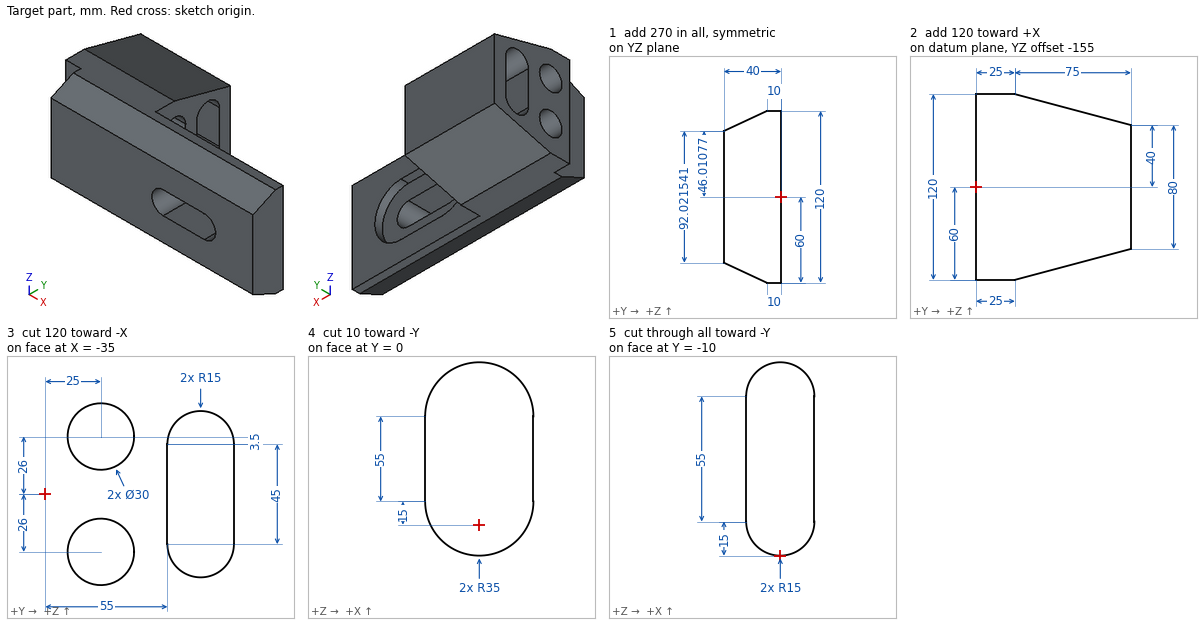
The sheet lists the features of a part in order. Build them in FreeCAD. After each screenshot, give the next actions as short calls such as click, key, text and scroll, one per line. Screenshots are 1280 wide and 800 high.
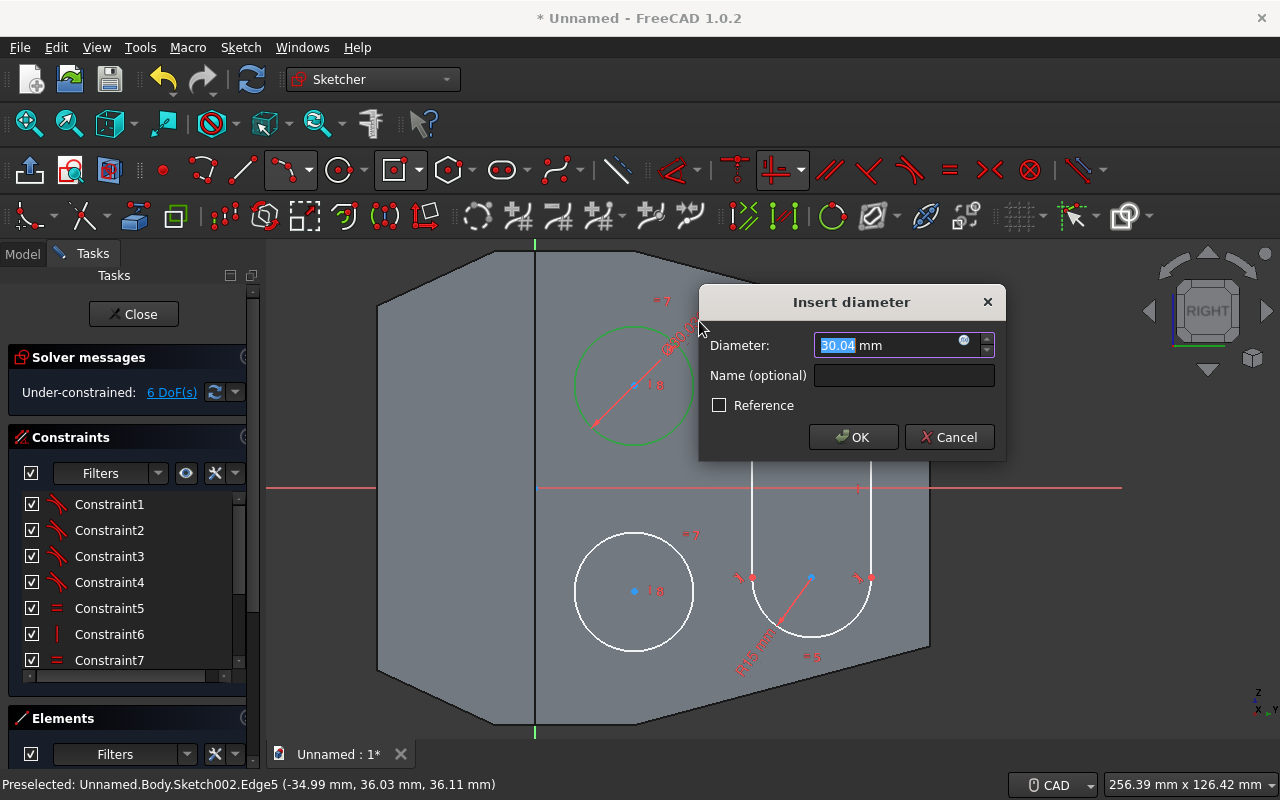
text(30)
key(Return)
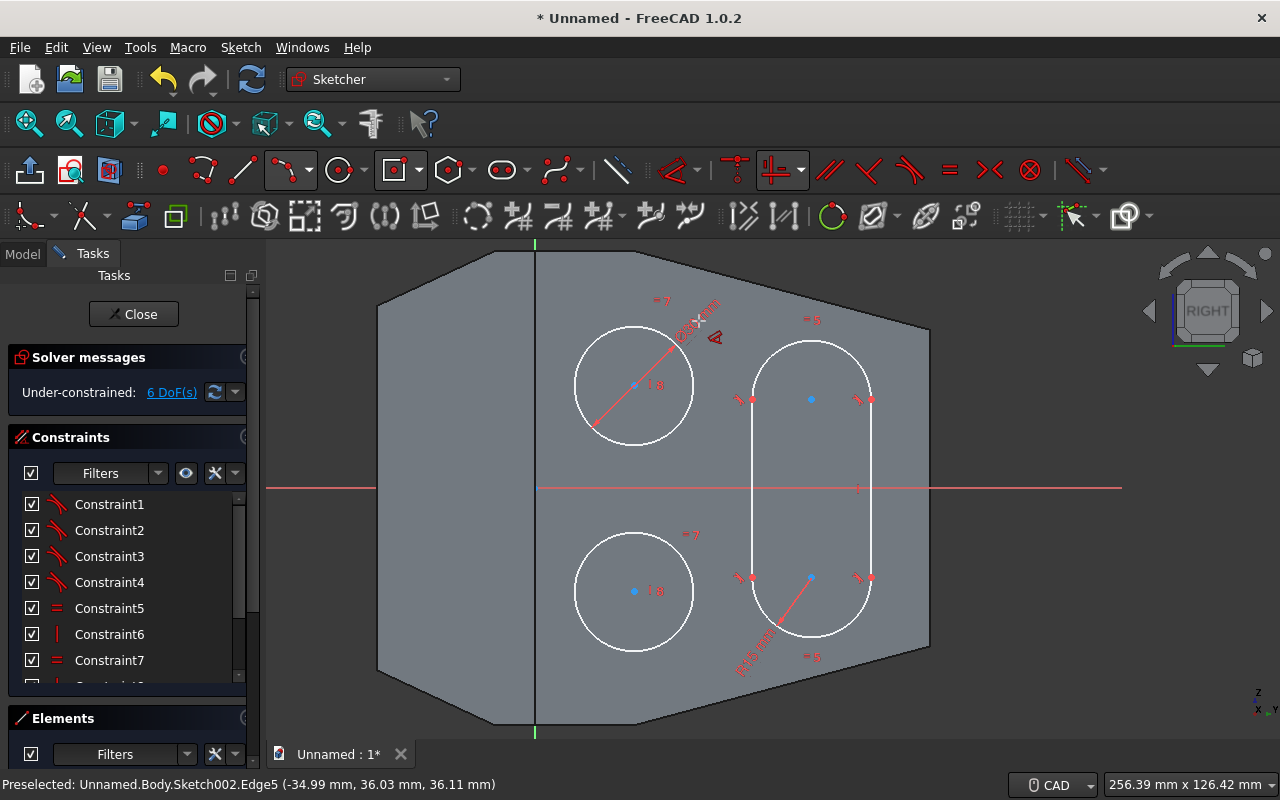
click(752, 525)
click(786, 448)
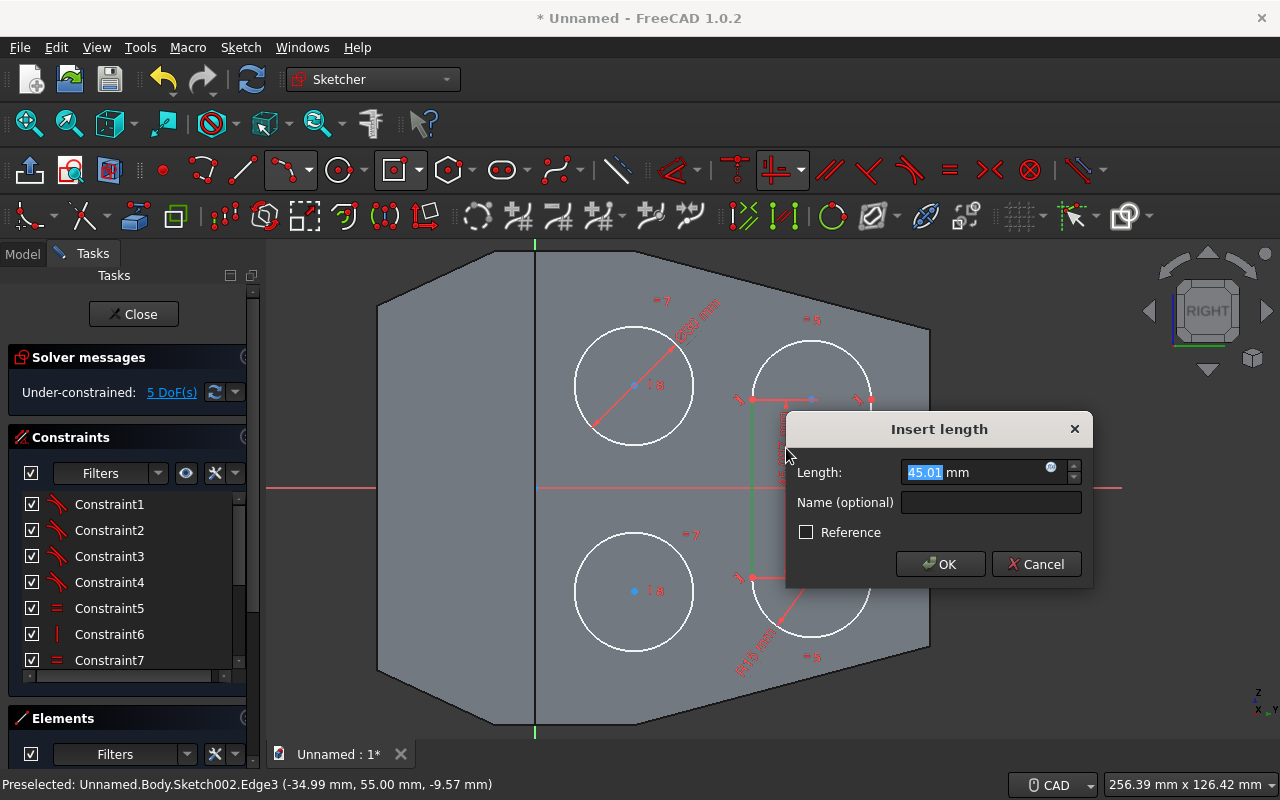
text(45)
key(Return)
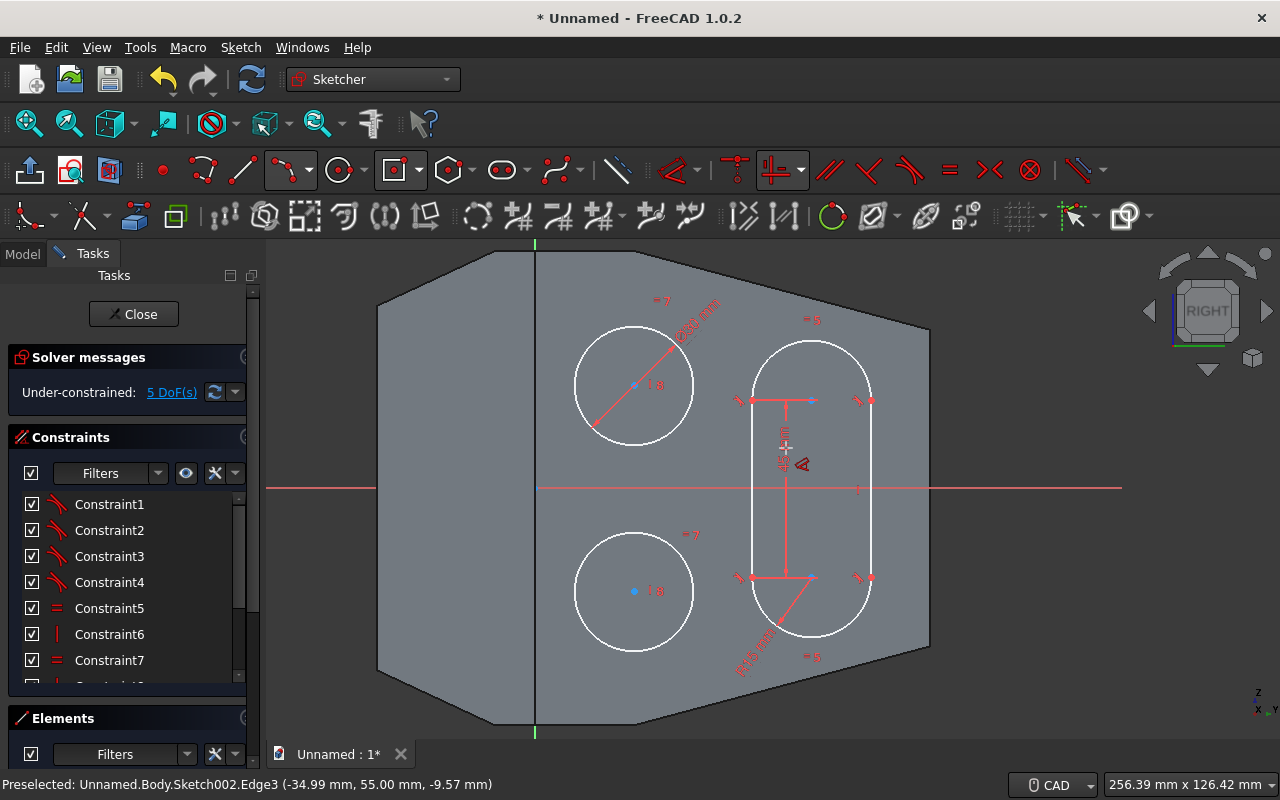
click(634, 386)
click(562, 352)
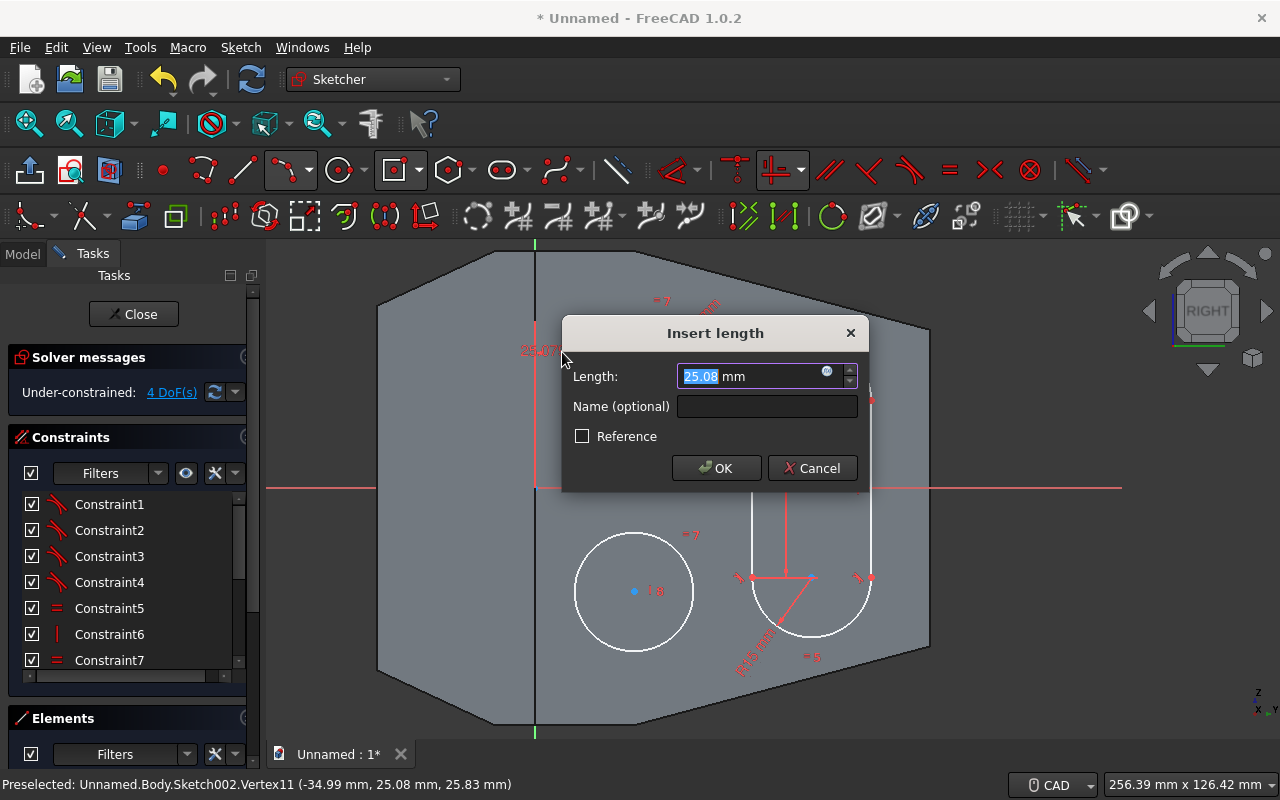
text(25)
key(Return)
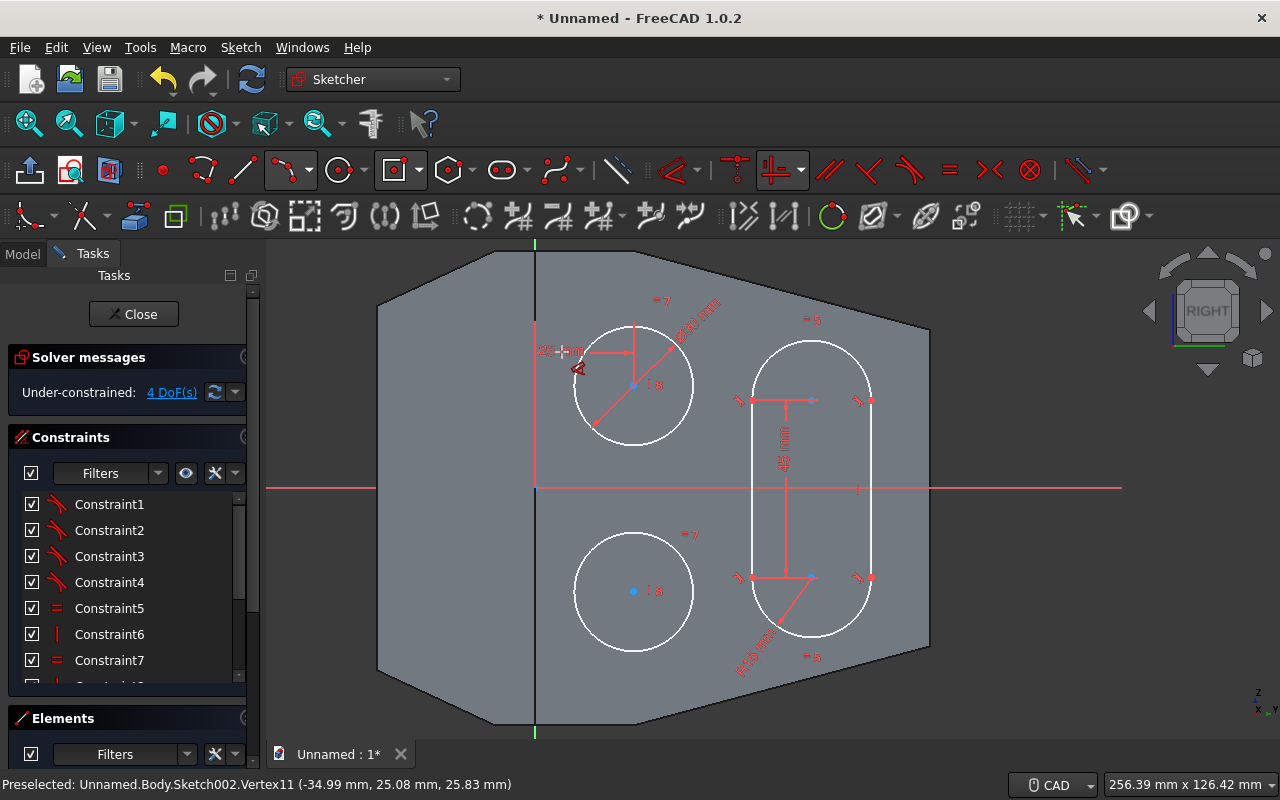
click(634, 386)
click(501, 437)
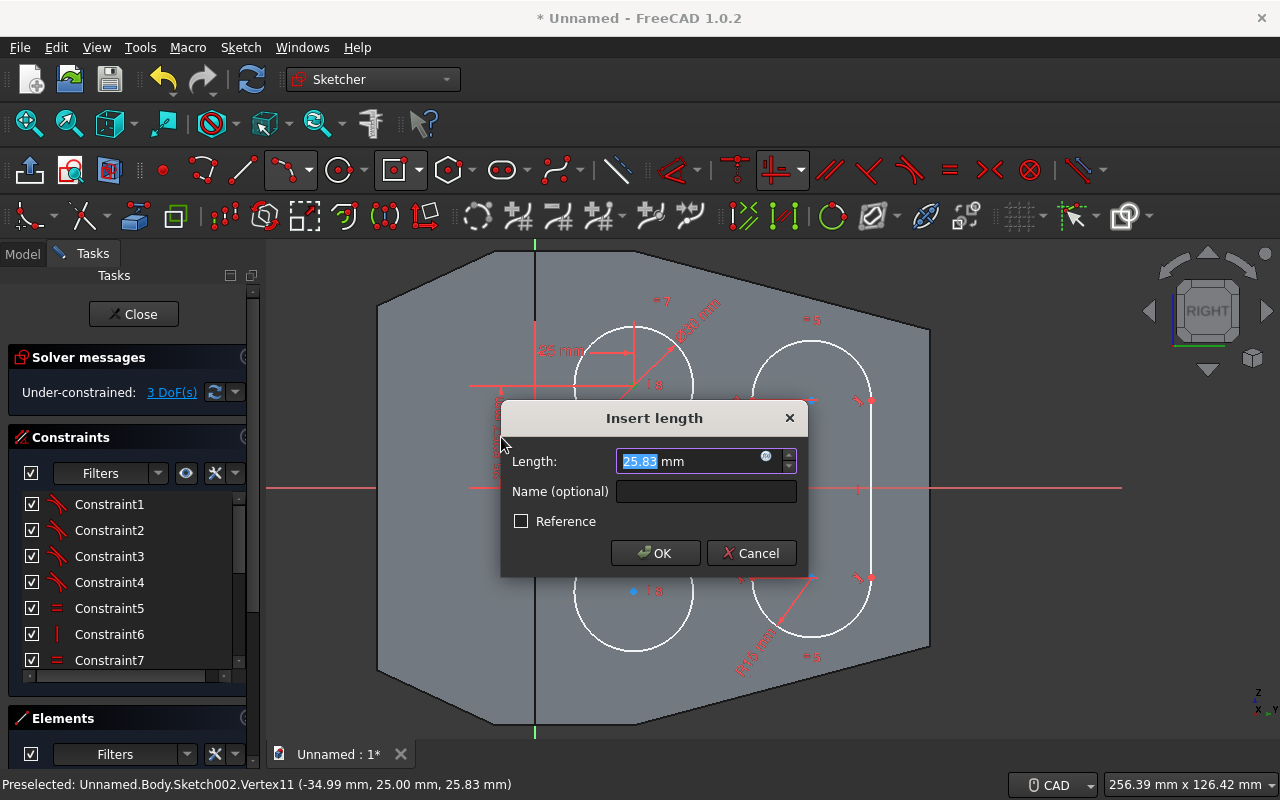
text(26)
key(Return)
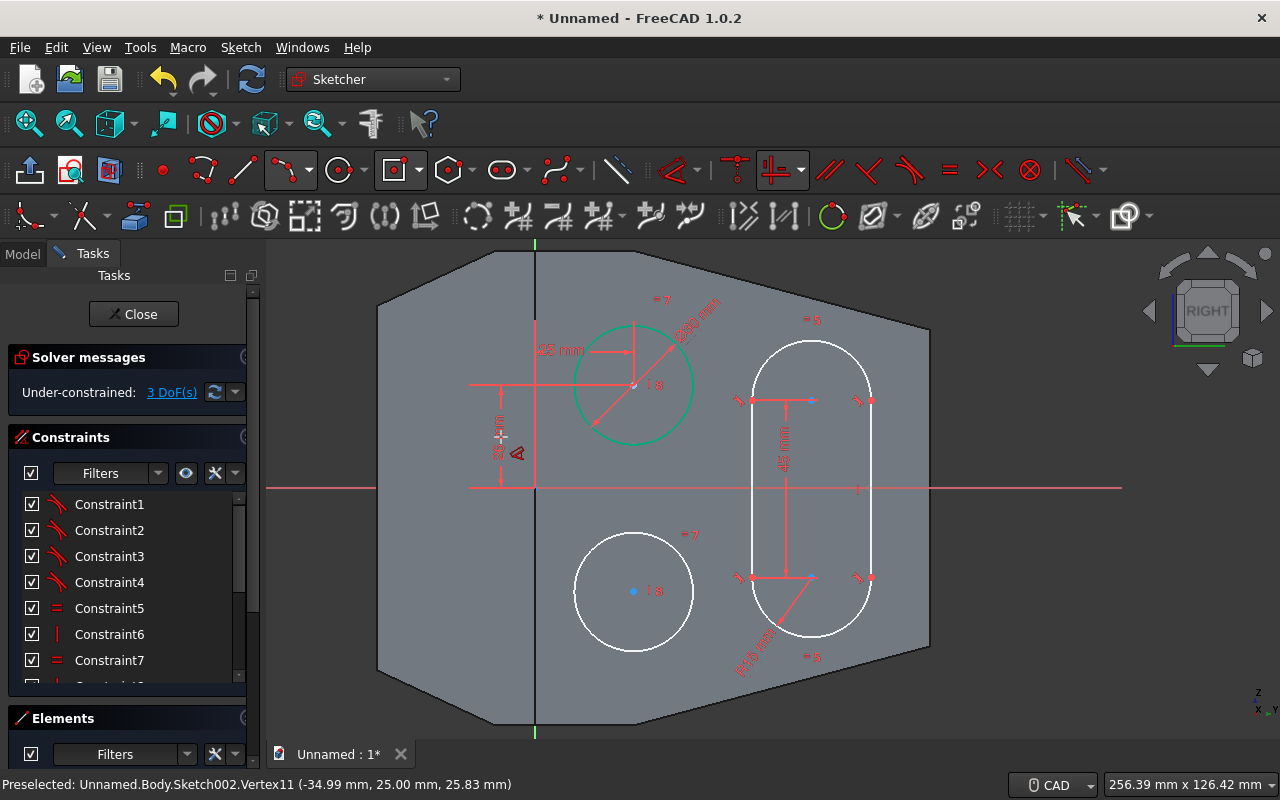
click(634, 592)
click(501, 540)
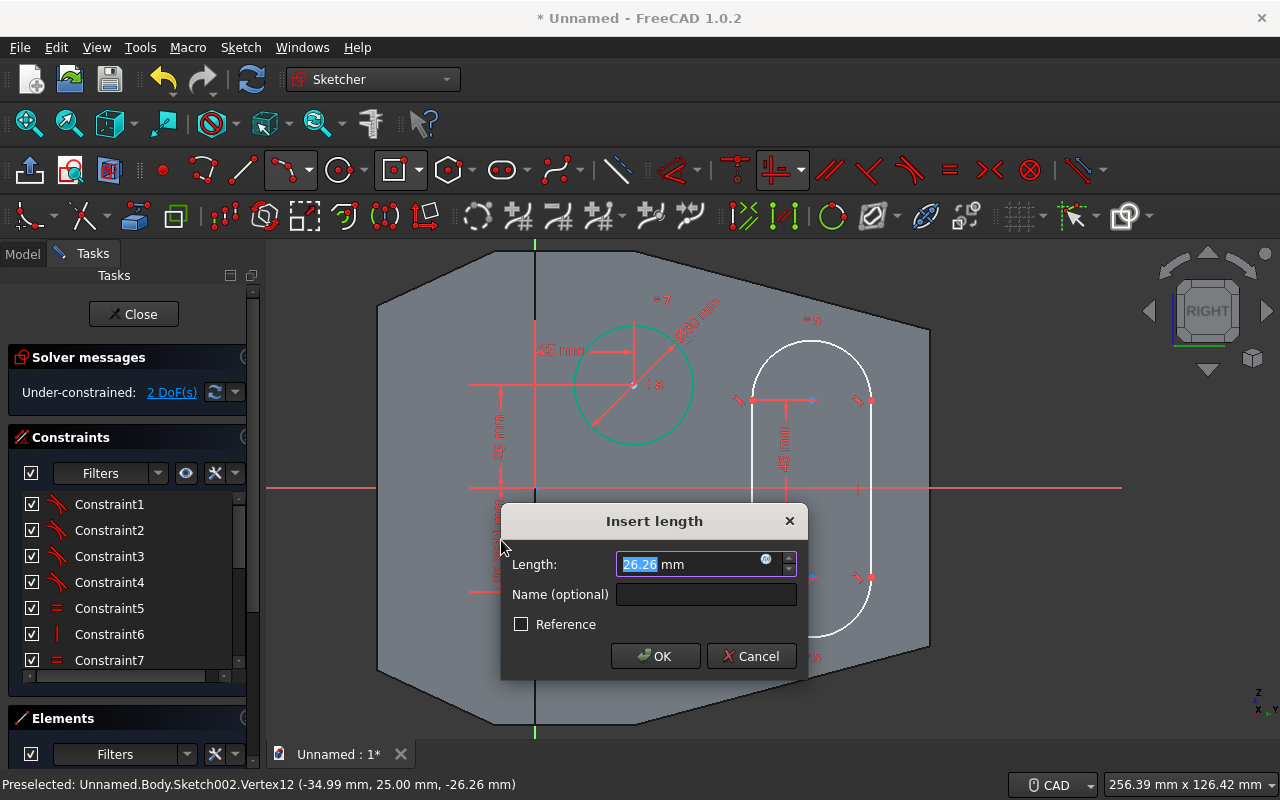
text(26)
key(Return)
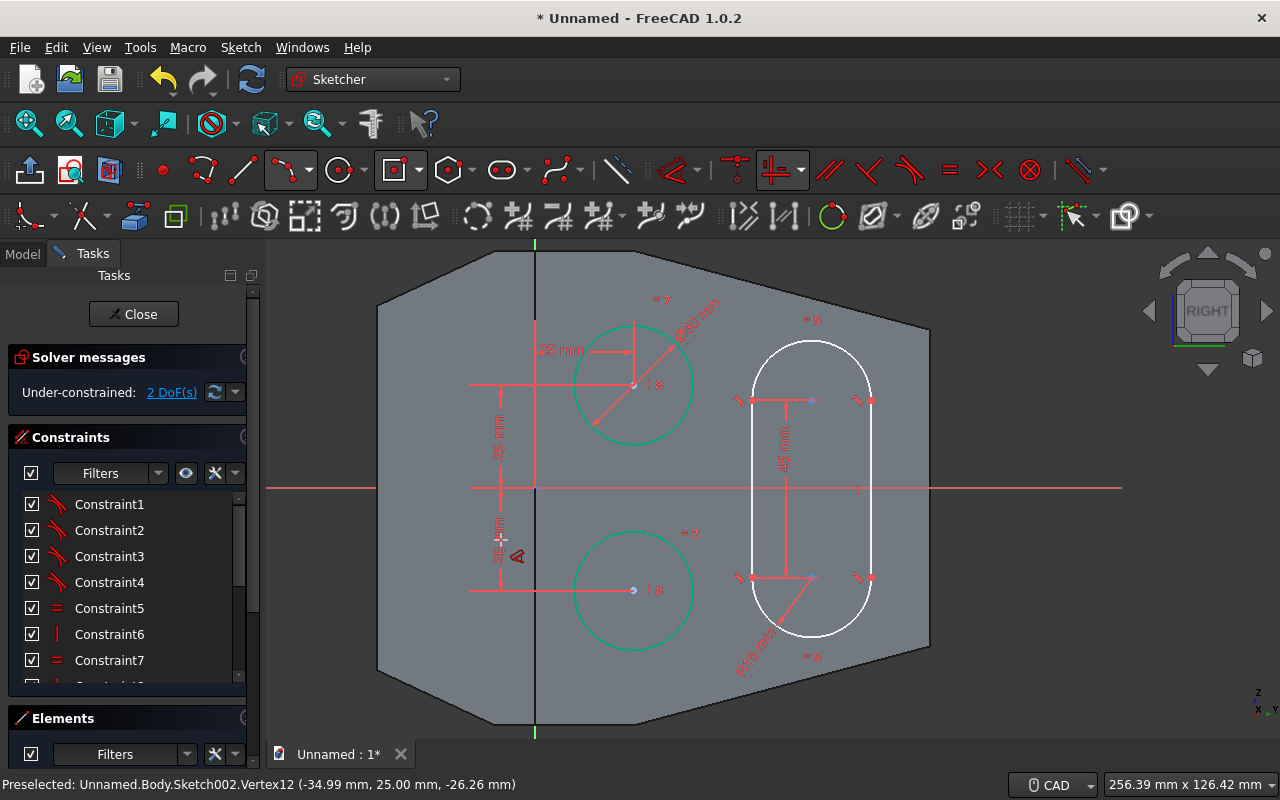
click(752, 578)
click(644, 612)